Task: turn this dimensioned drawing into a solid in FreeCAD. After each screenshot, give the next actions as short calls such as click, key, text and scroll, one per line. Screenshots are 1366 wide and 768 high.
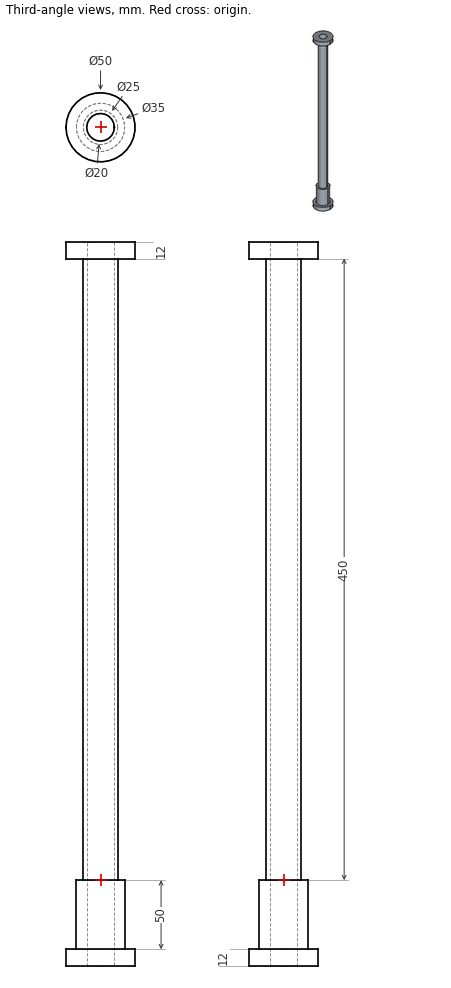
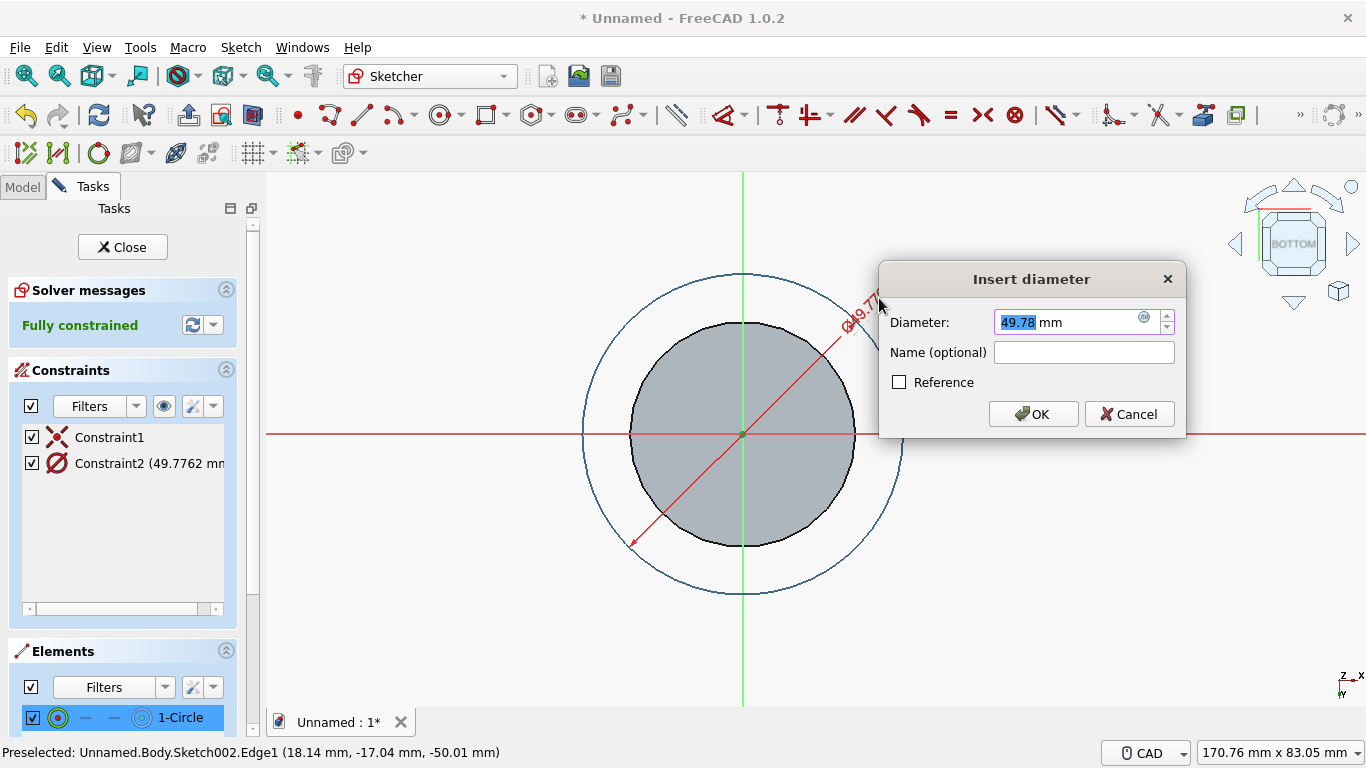
text(50)
key(Return)
key(Escape)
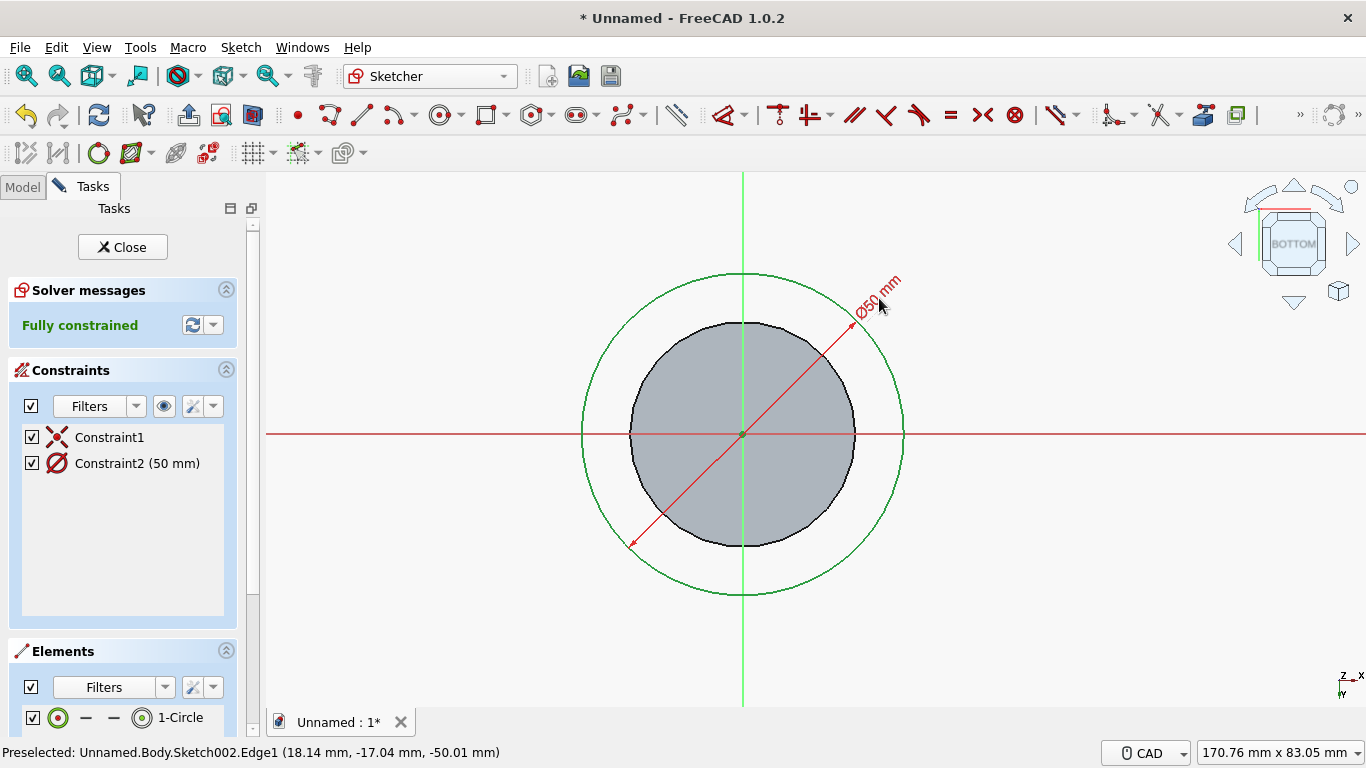
click(123, 247)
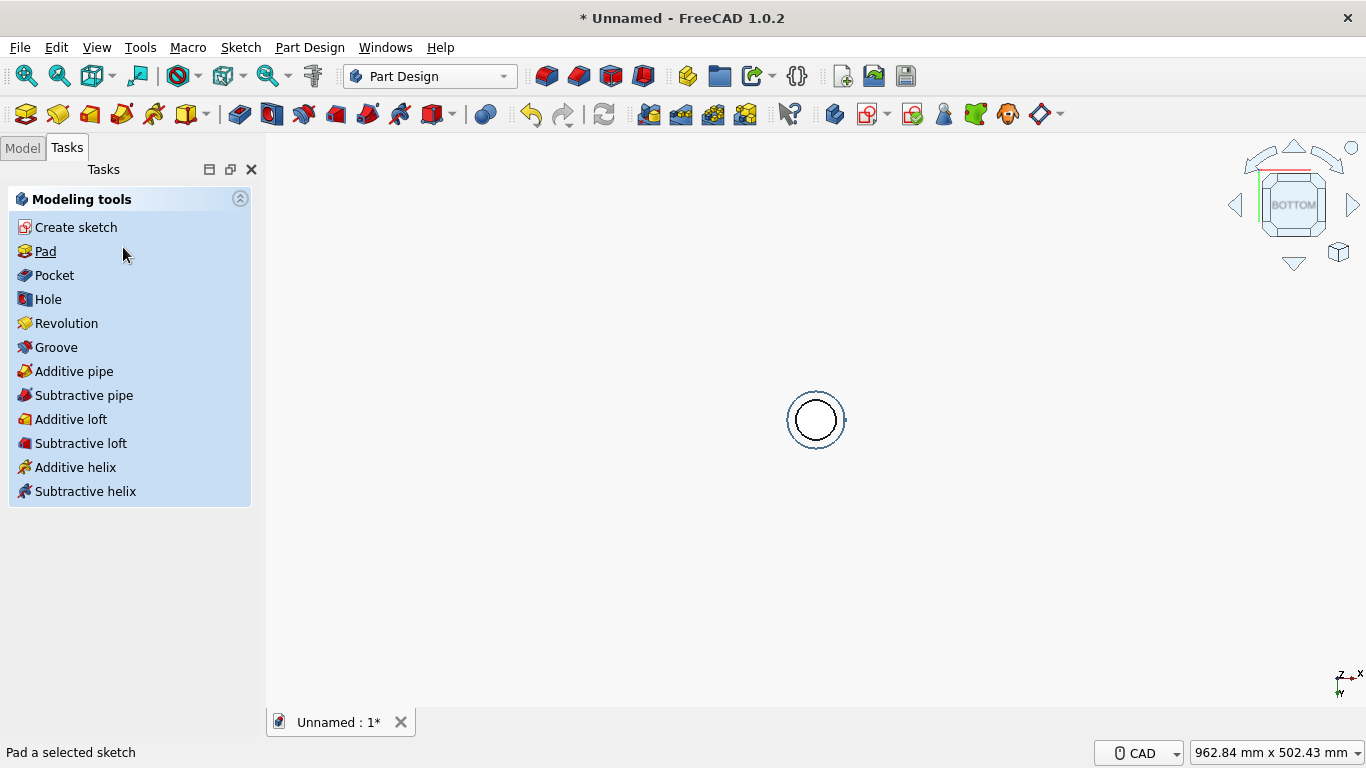
click(26, 114)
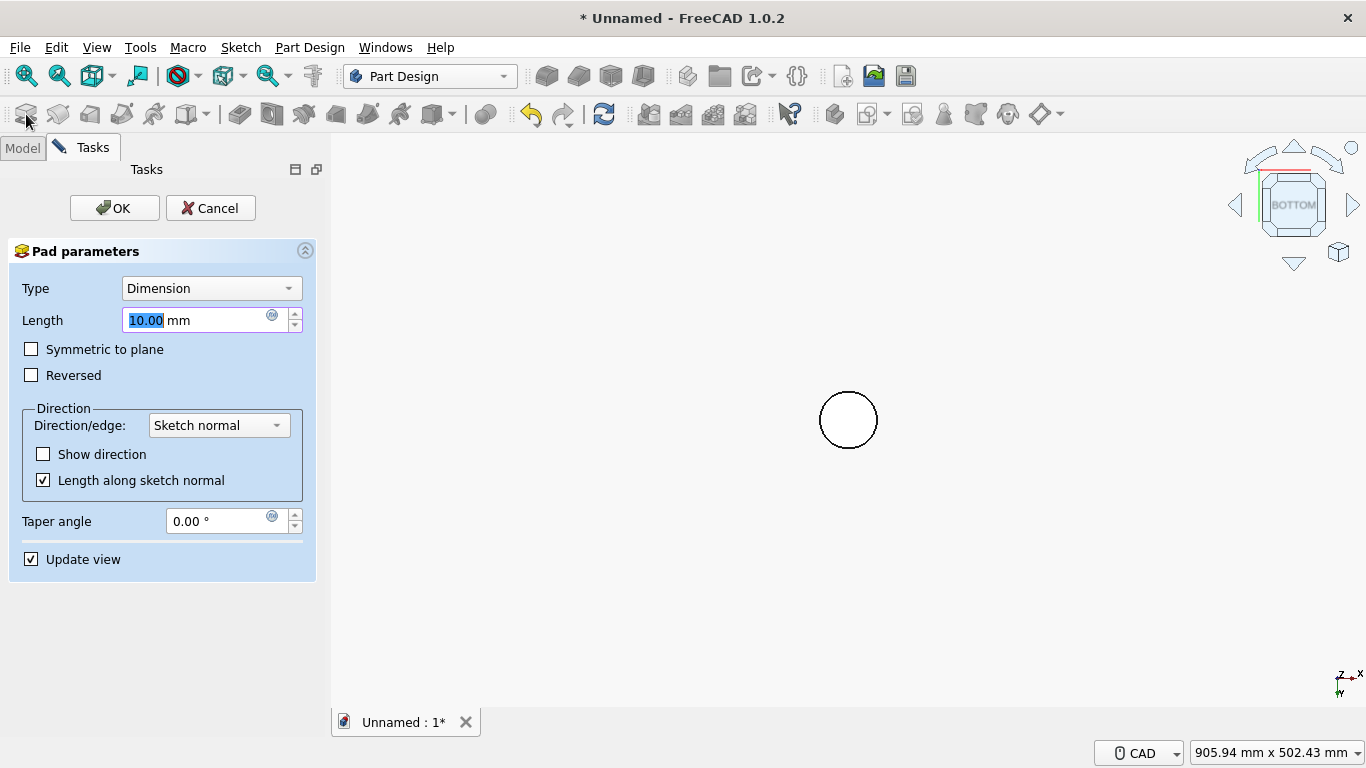
text(12)
key(Tab)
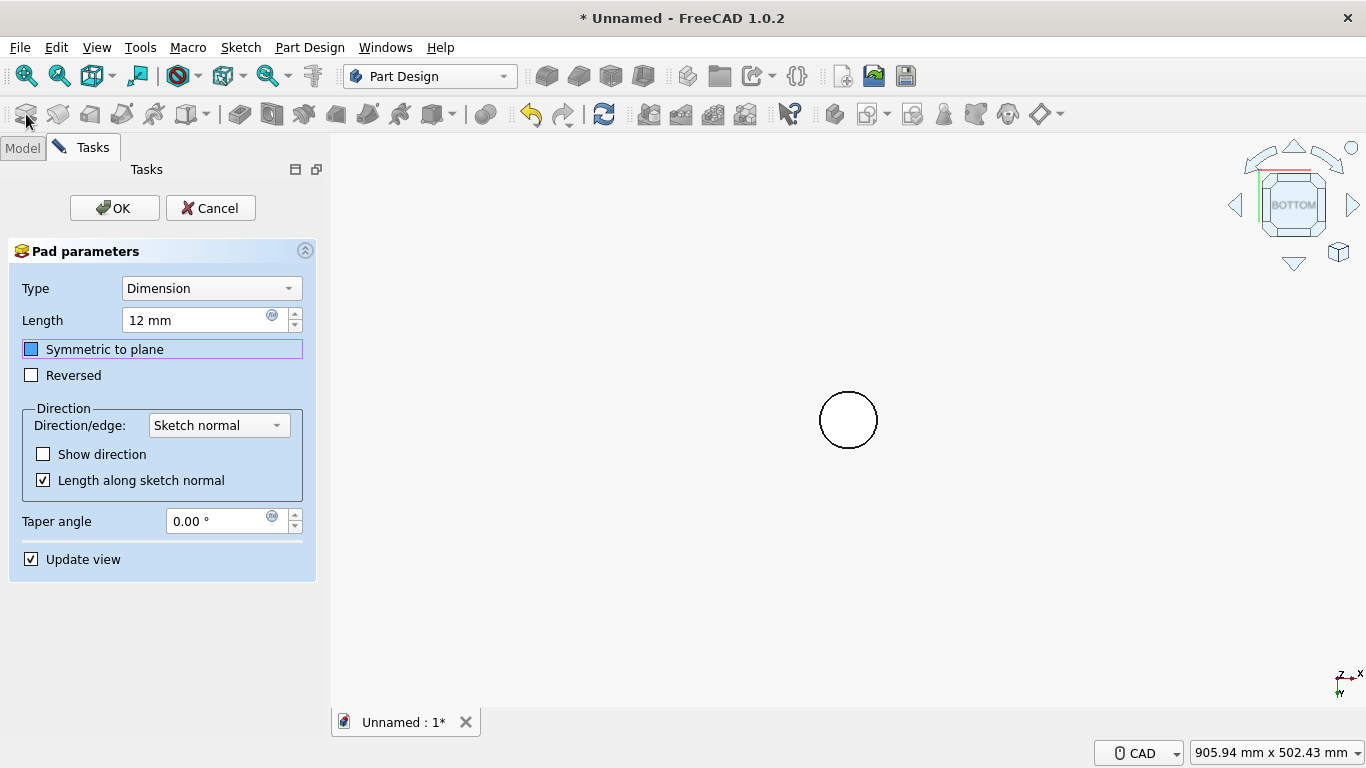
click(115, 208)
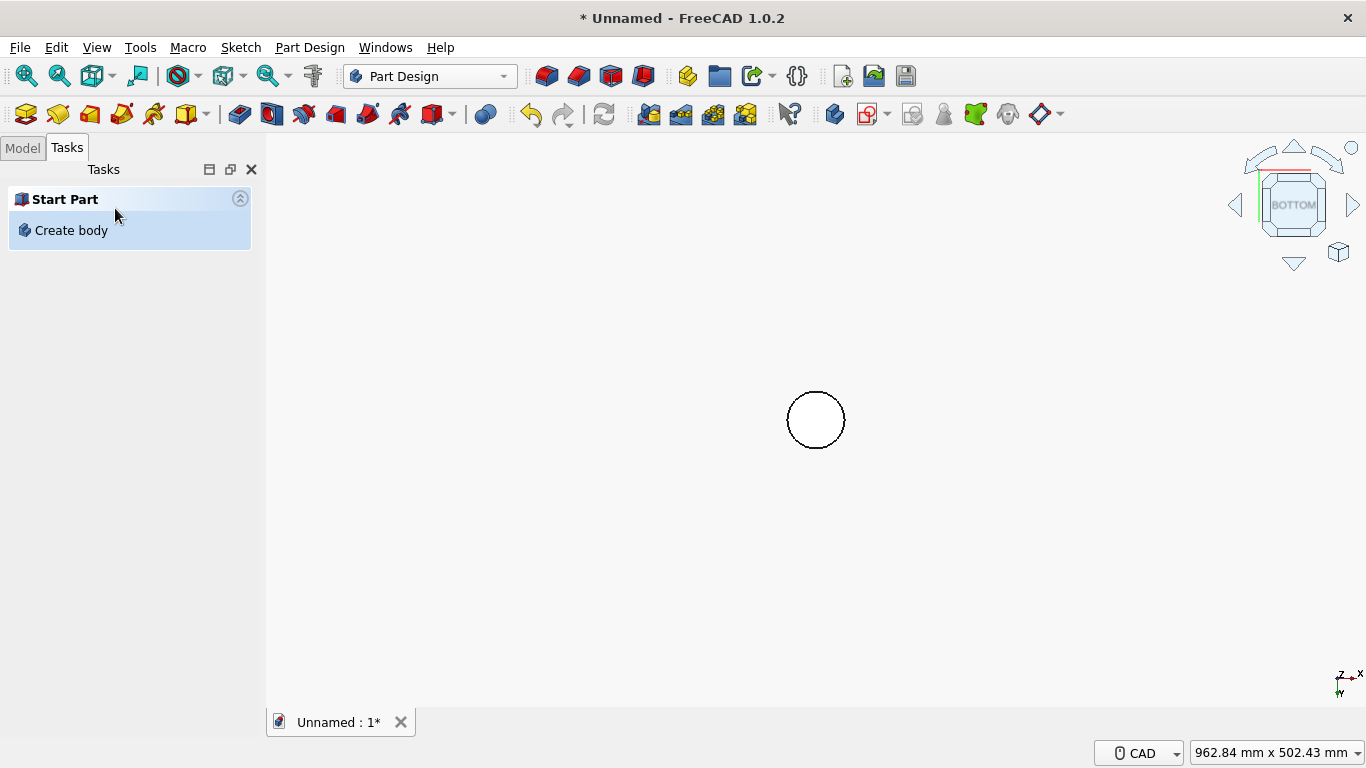
click(28, 76)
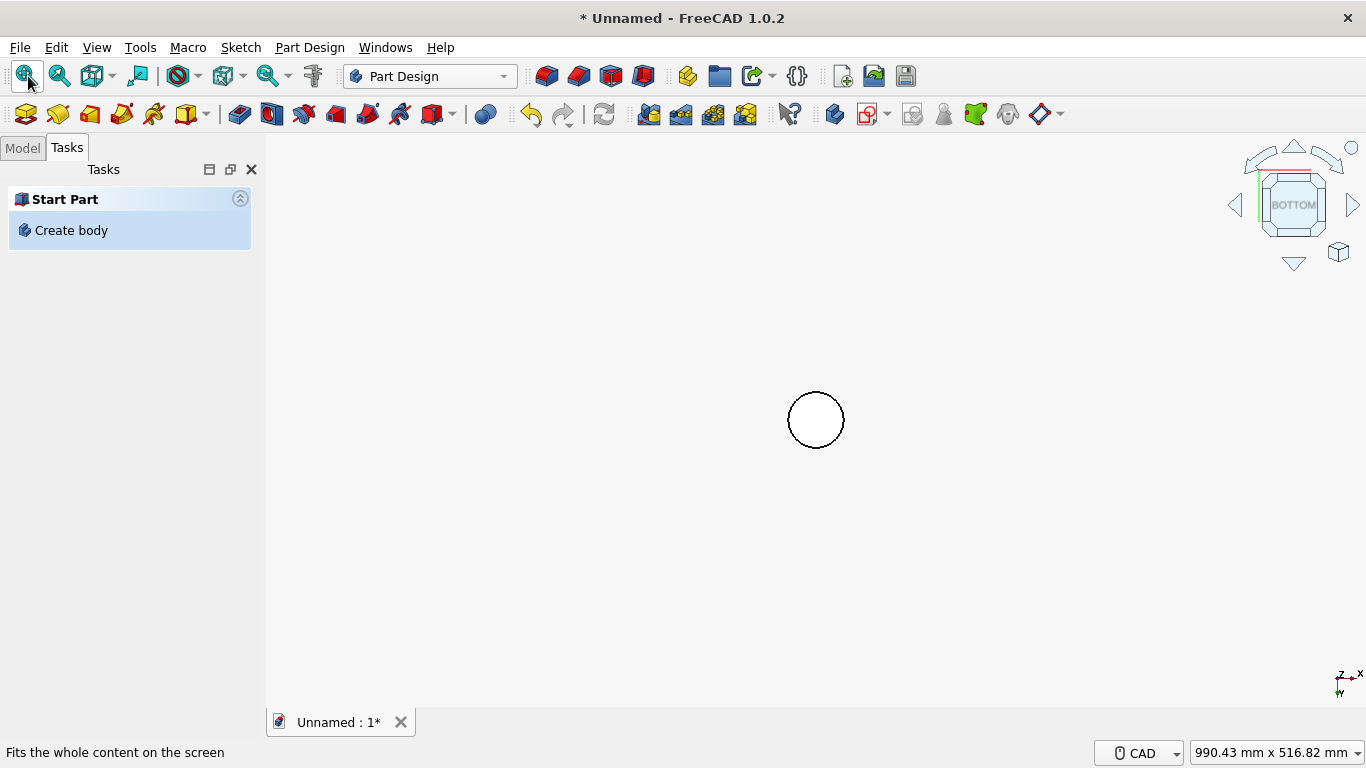
click(23, 147)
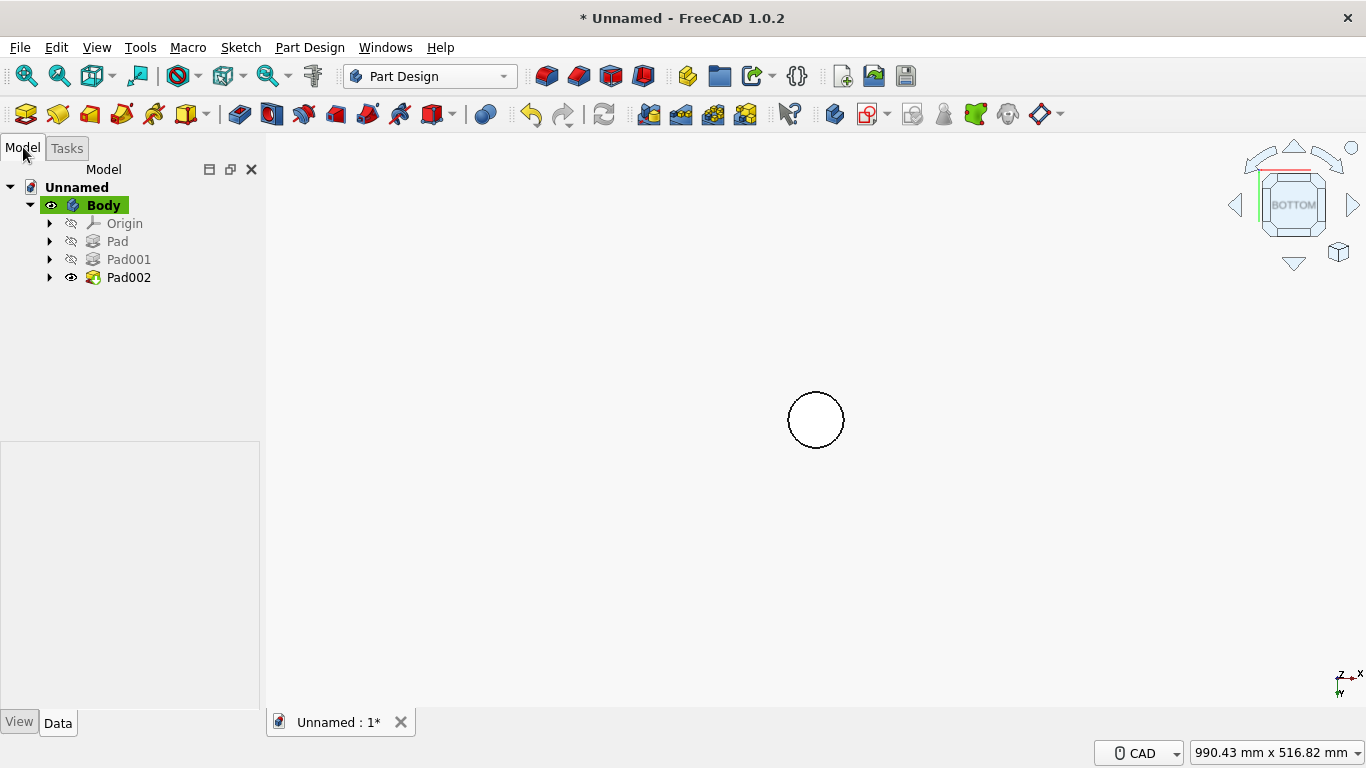
click(50, 223)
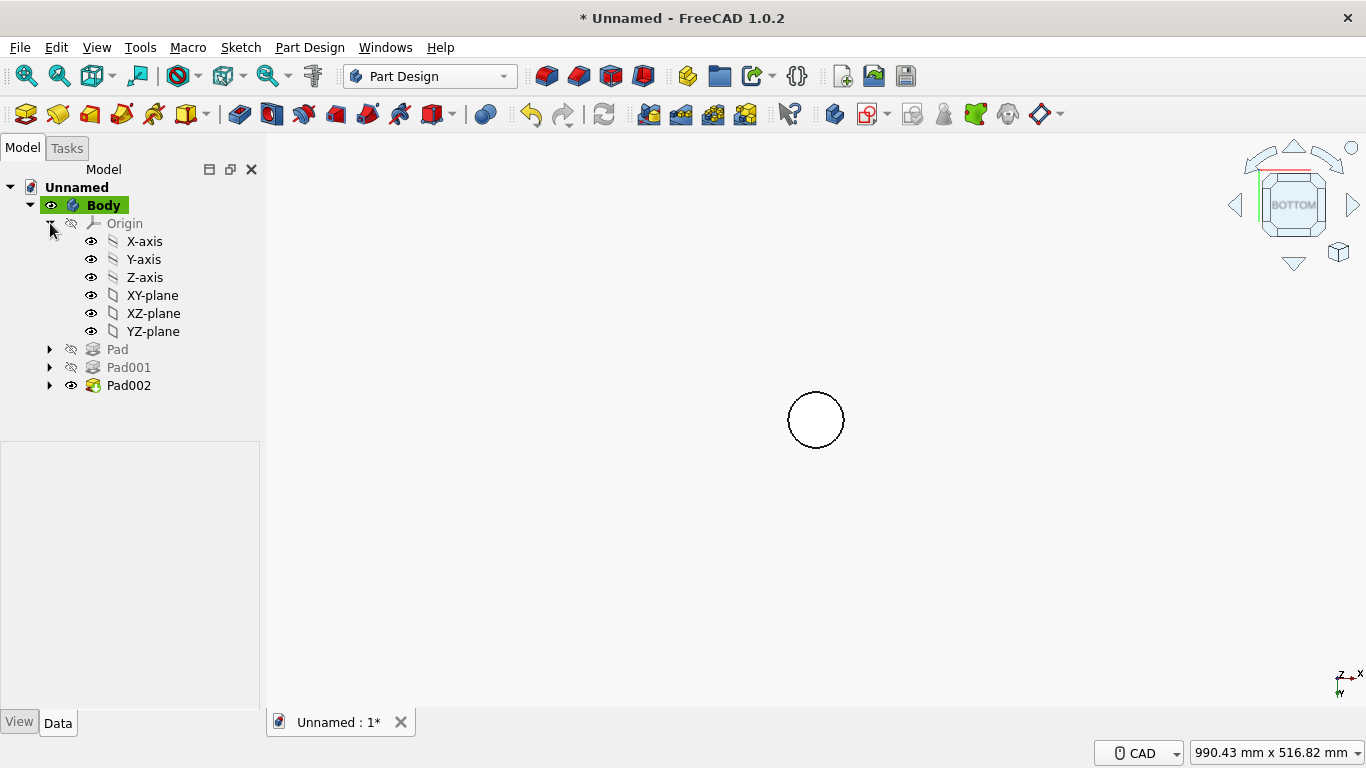
click(136, 295)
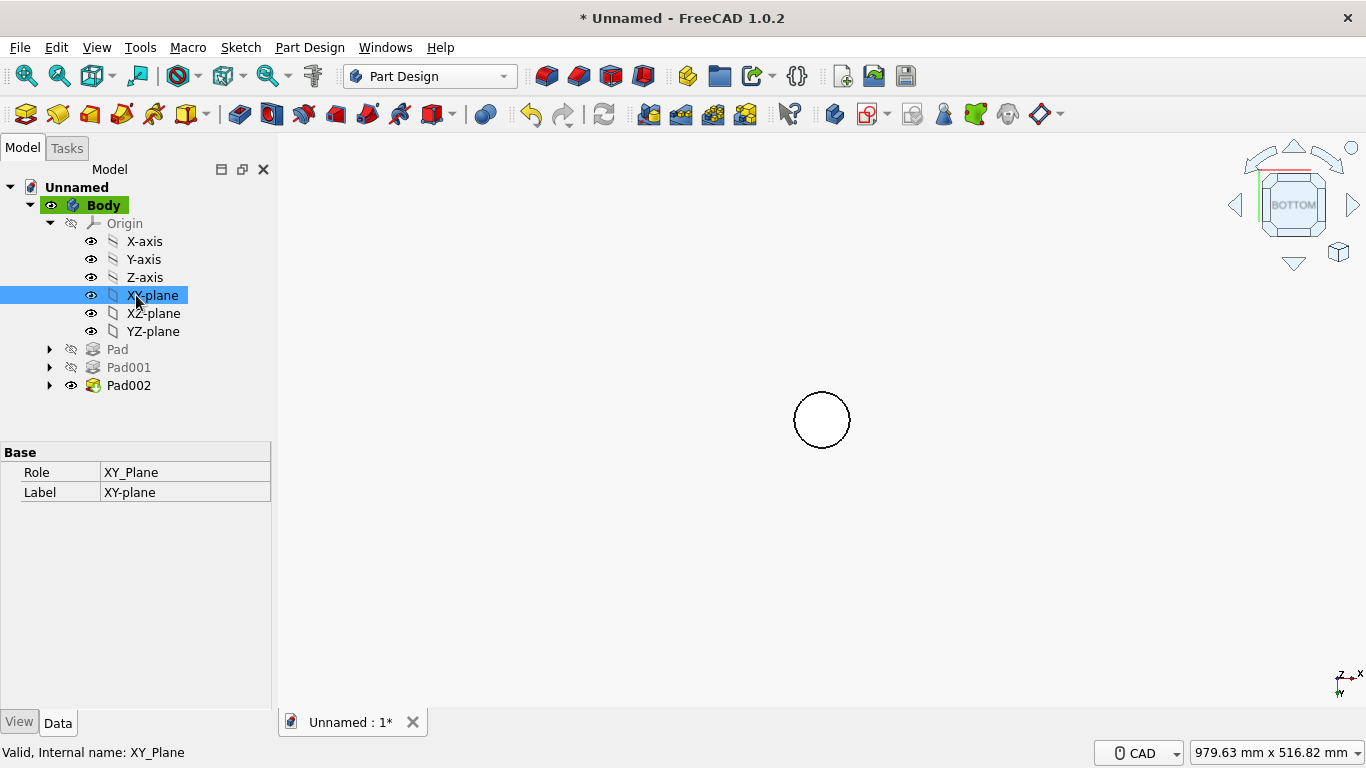
click(1040, 114)